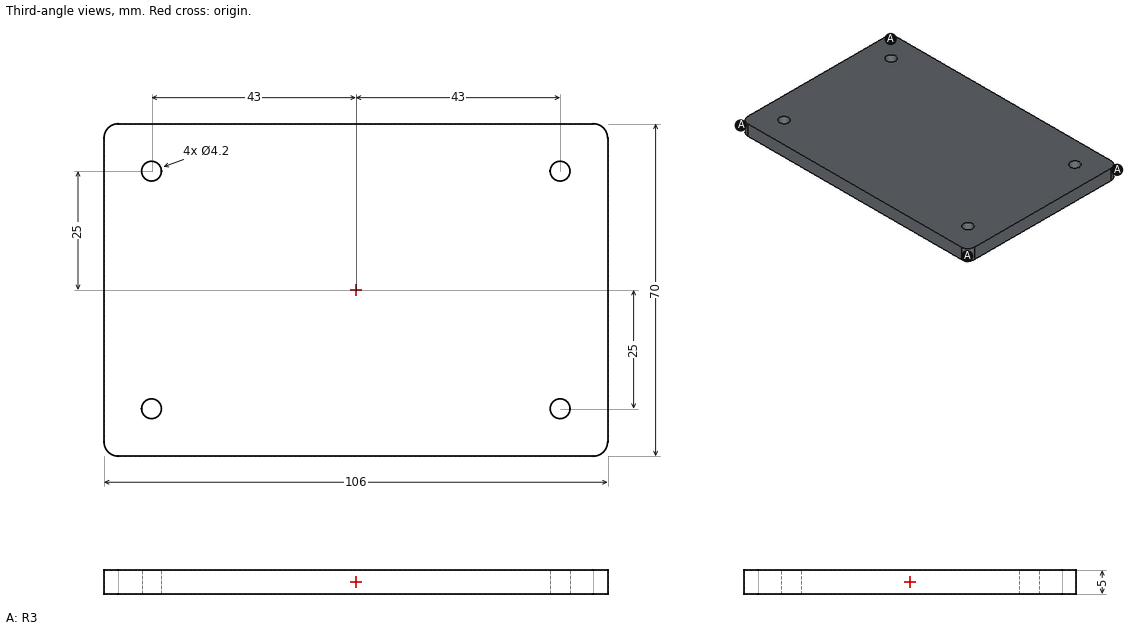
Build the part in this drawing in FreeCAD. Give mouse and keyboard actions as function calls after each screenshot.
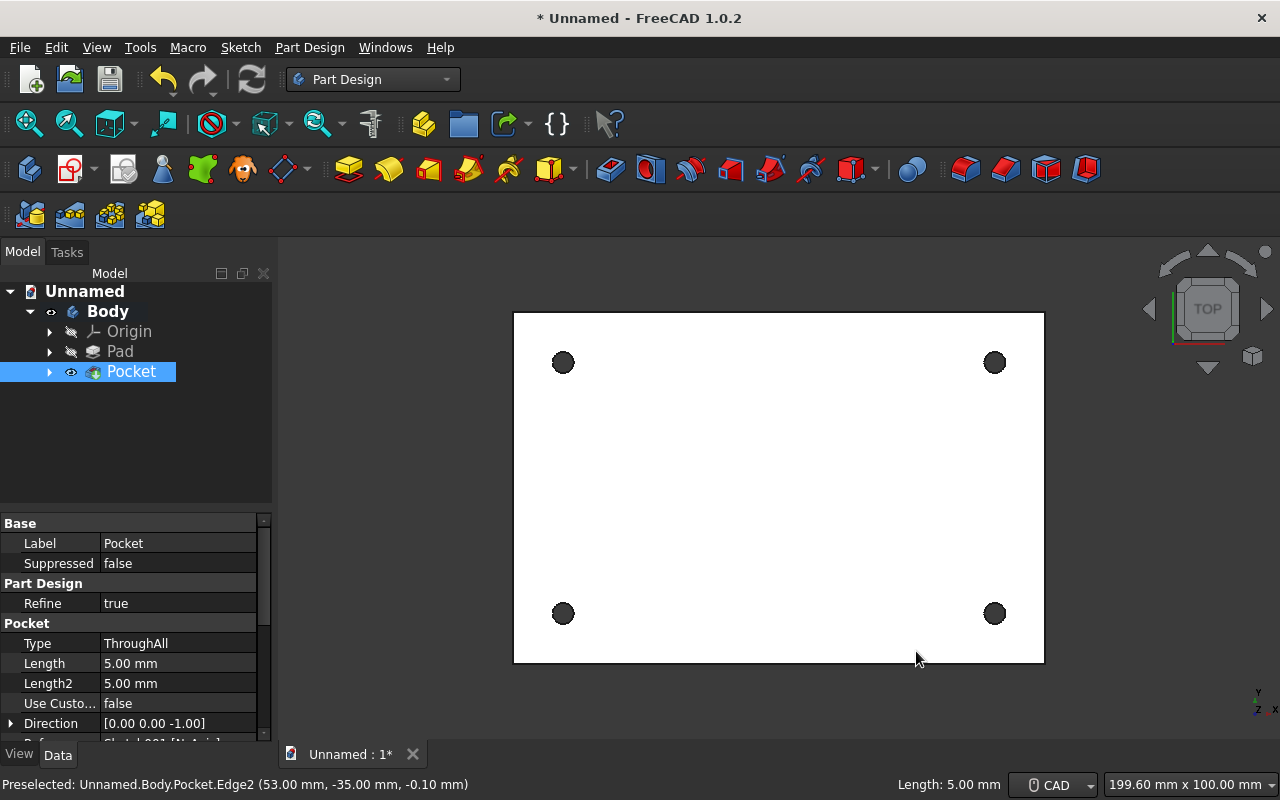
key(1)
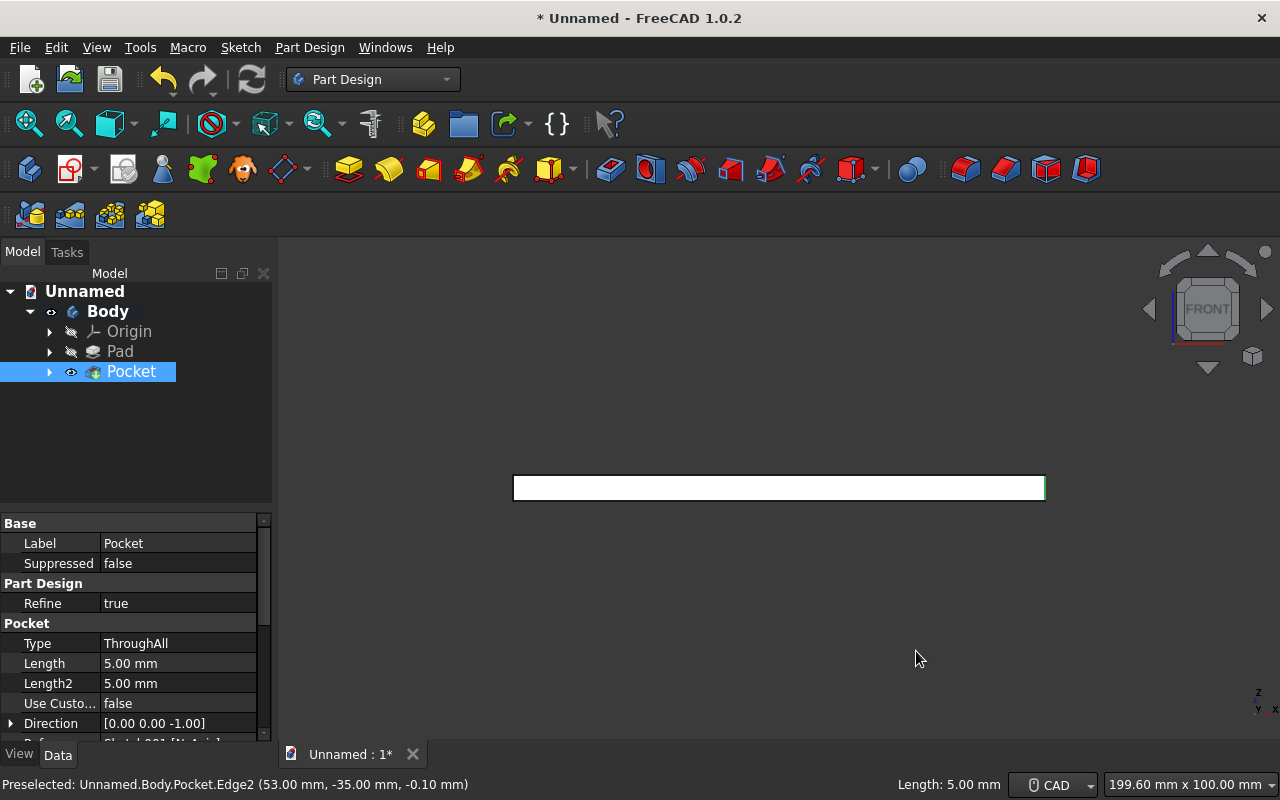
click(513, 487, ctrl)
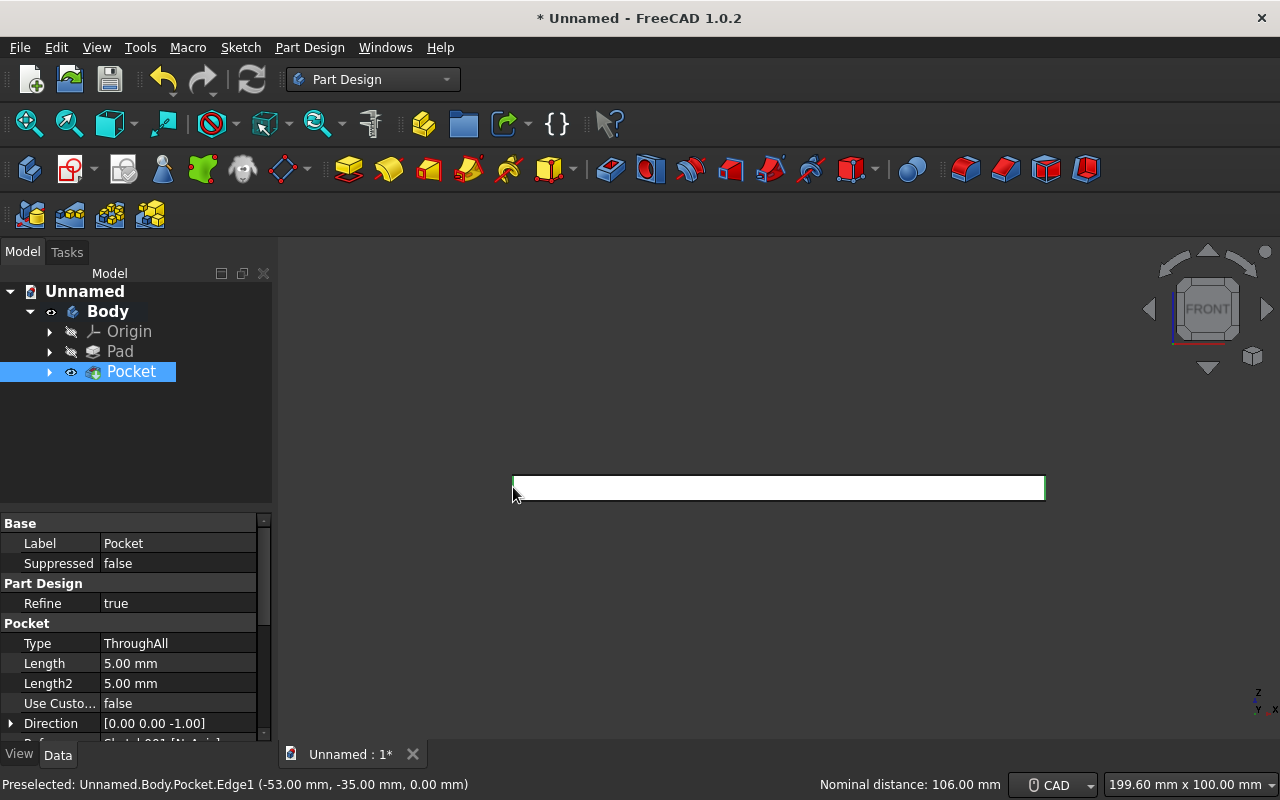
key(3)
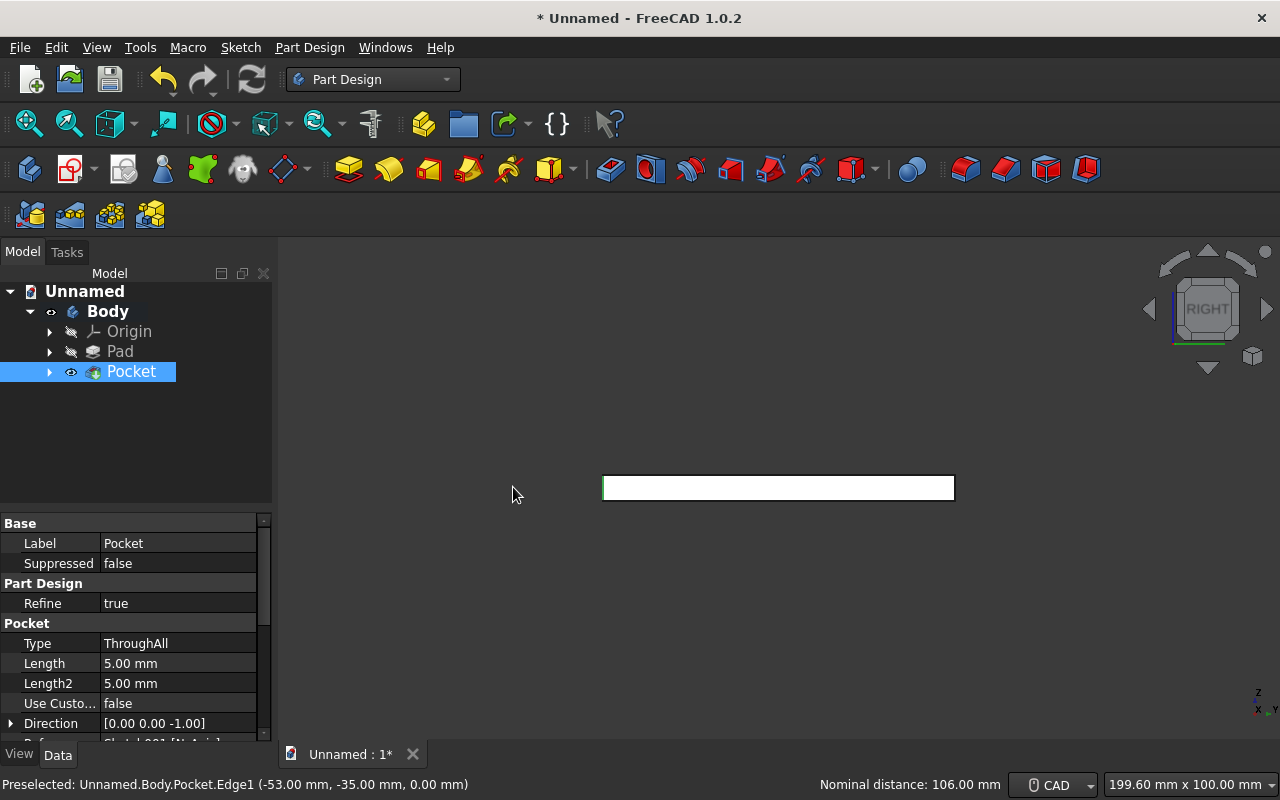
click(30, 124)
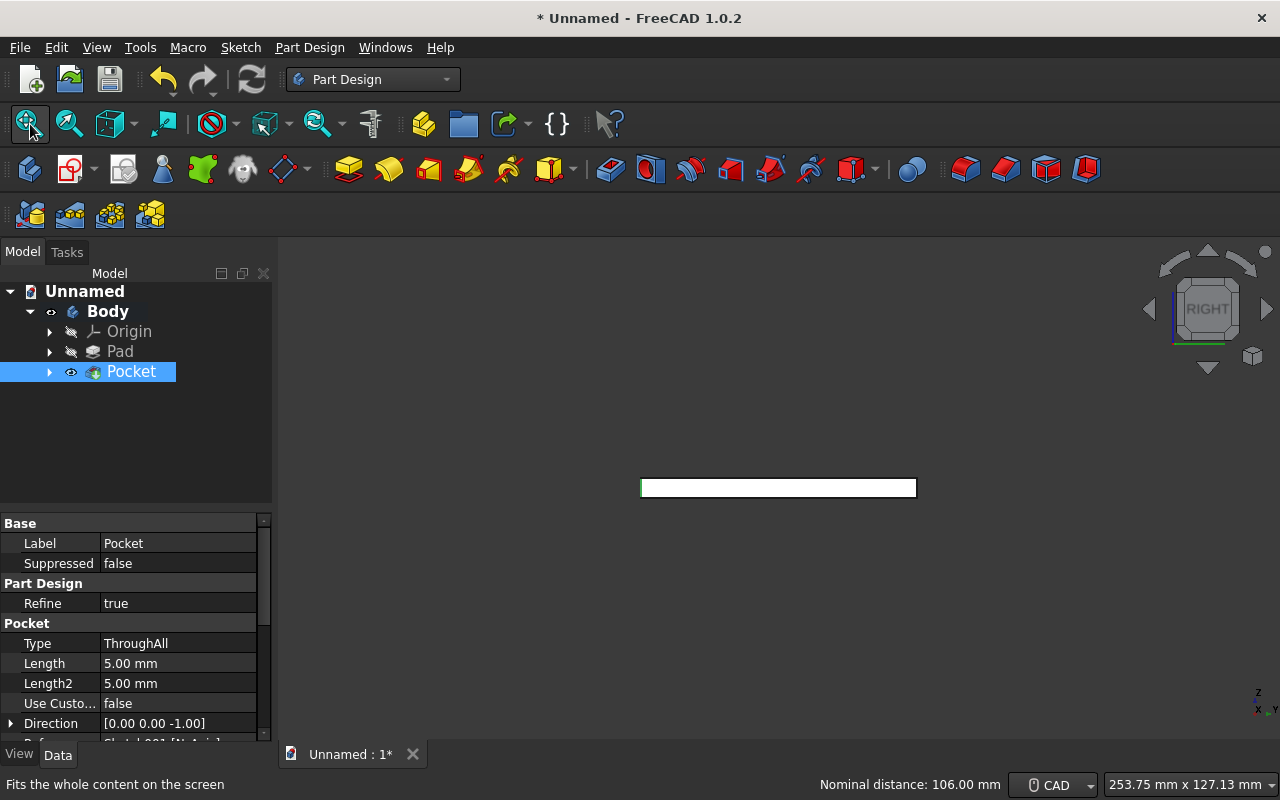
click(917, 487, ctrl)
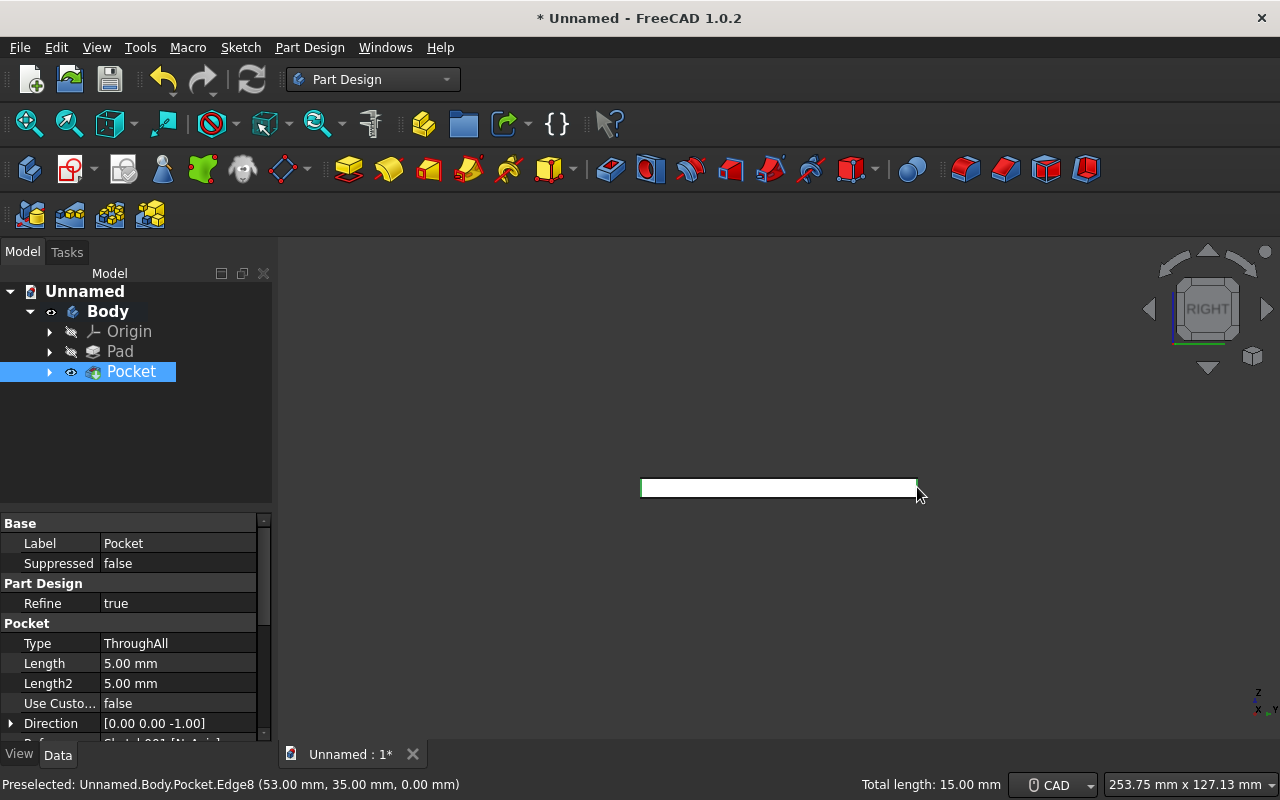
scroll(917, 487, up, 4)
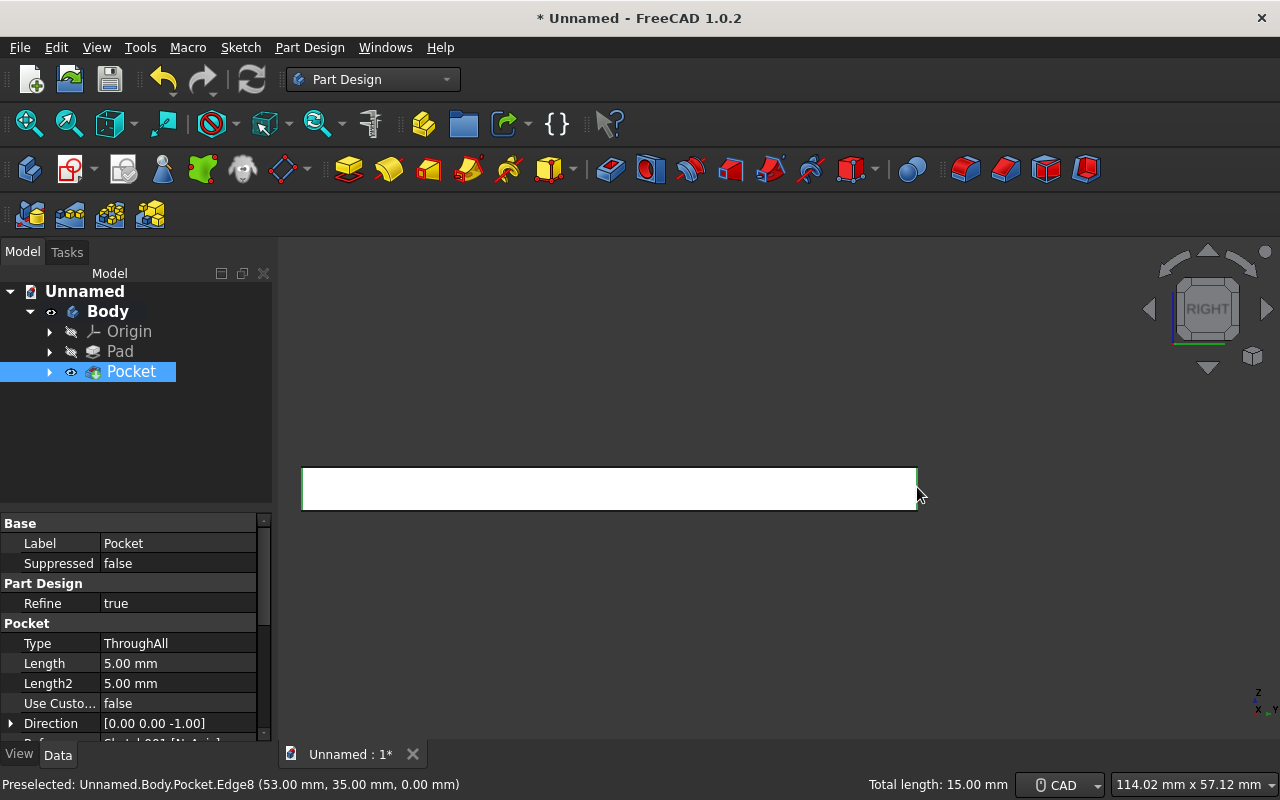
click(30, 124)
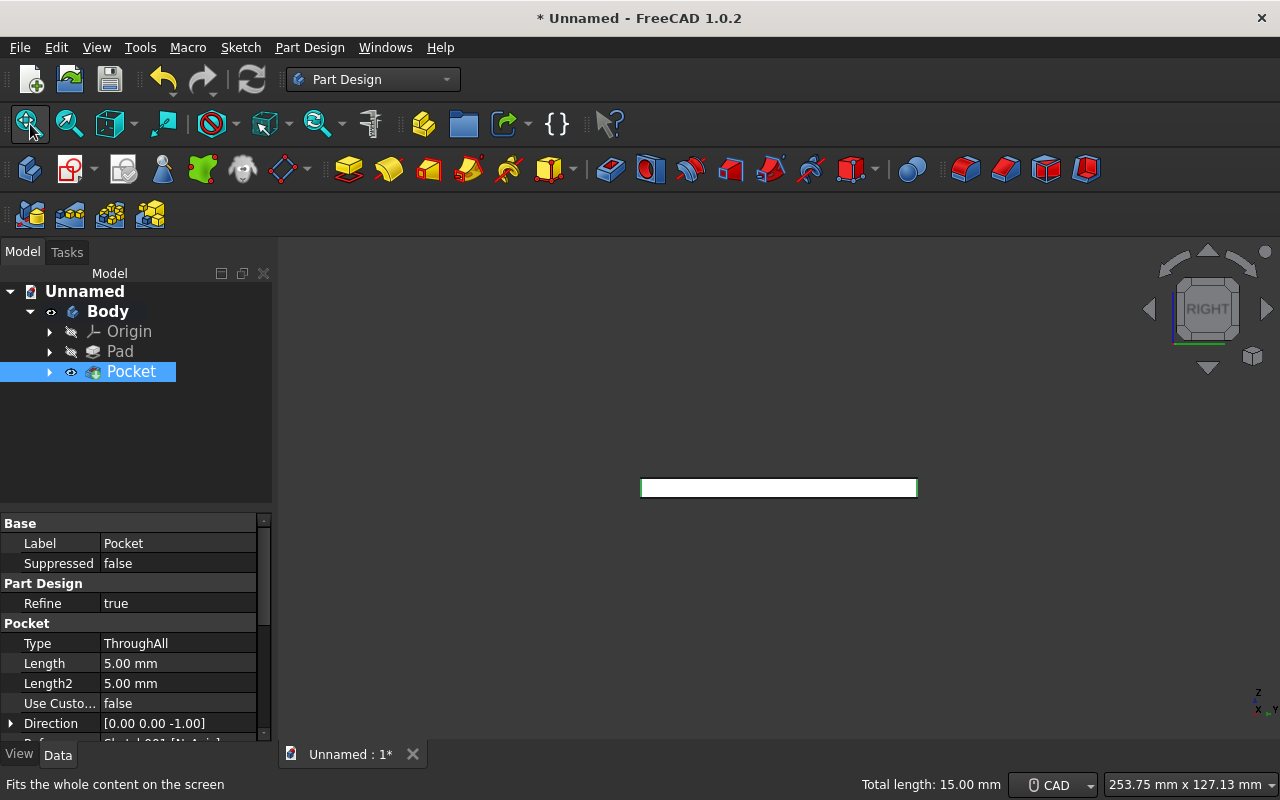
key(5)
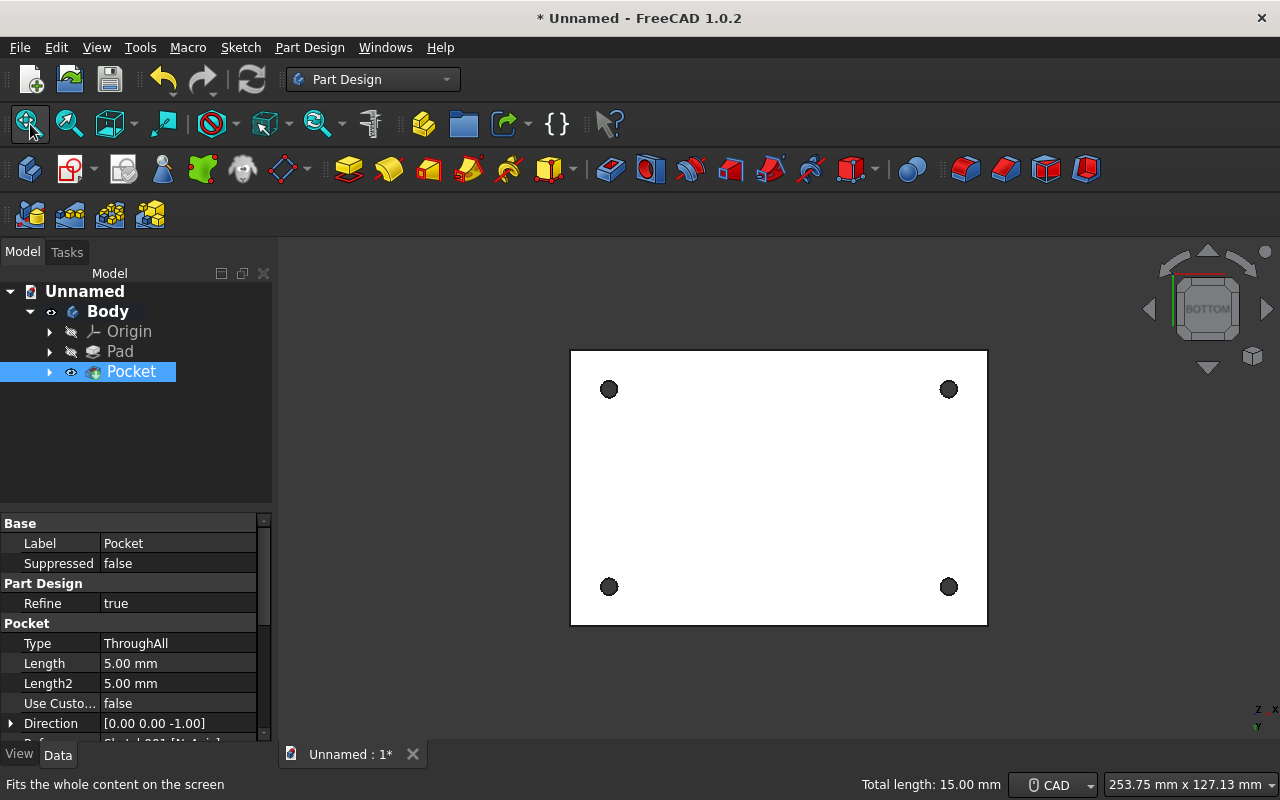
scroll(570, 625, up, 4)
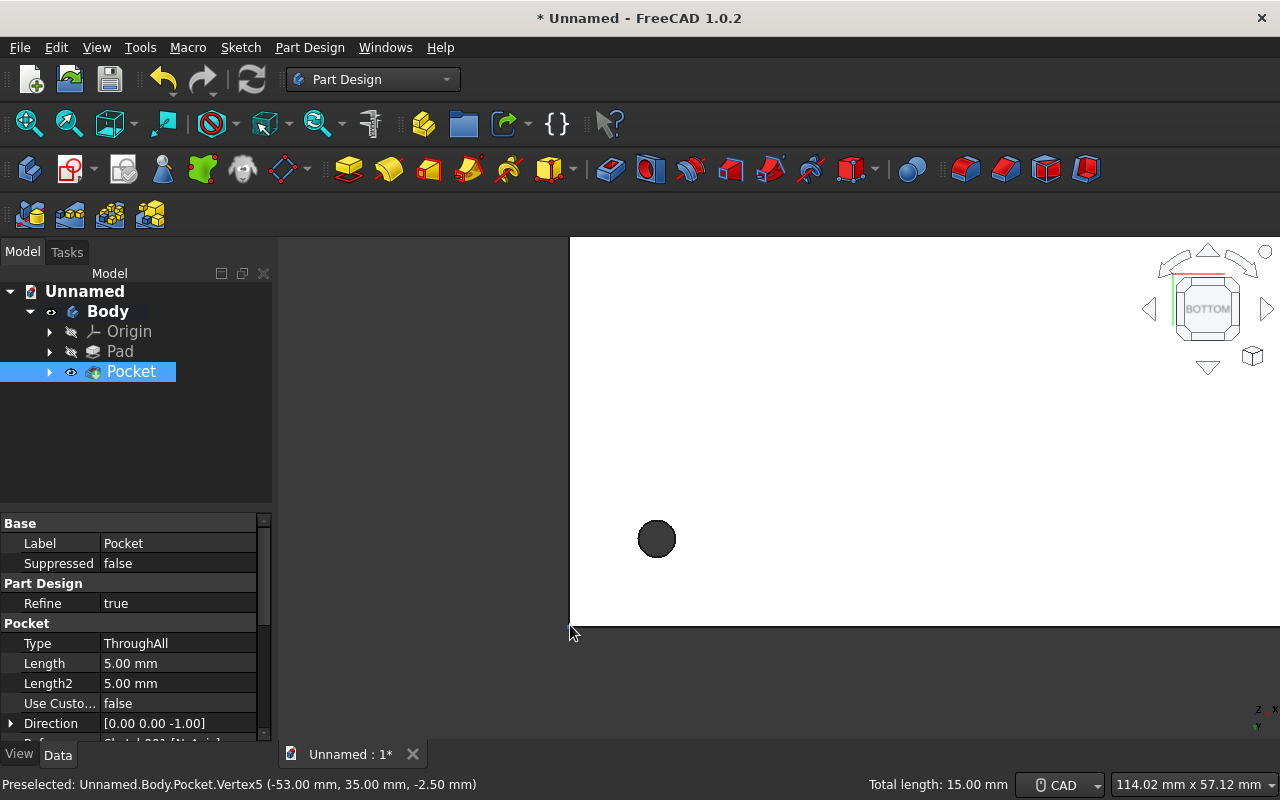
click(30, 124)